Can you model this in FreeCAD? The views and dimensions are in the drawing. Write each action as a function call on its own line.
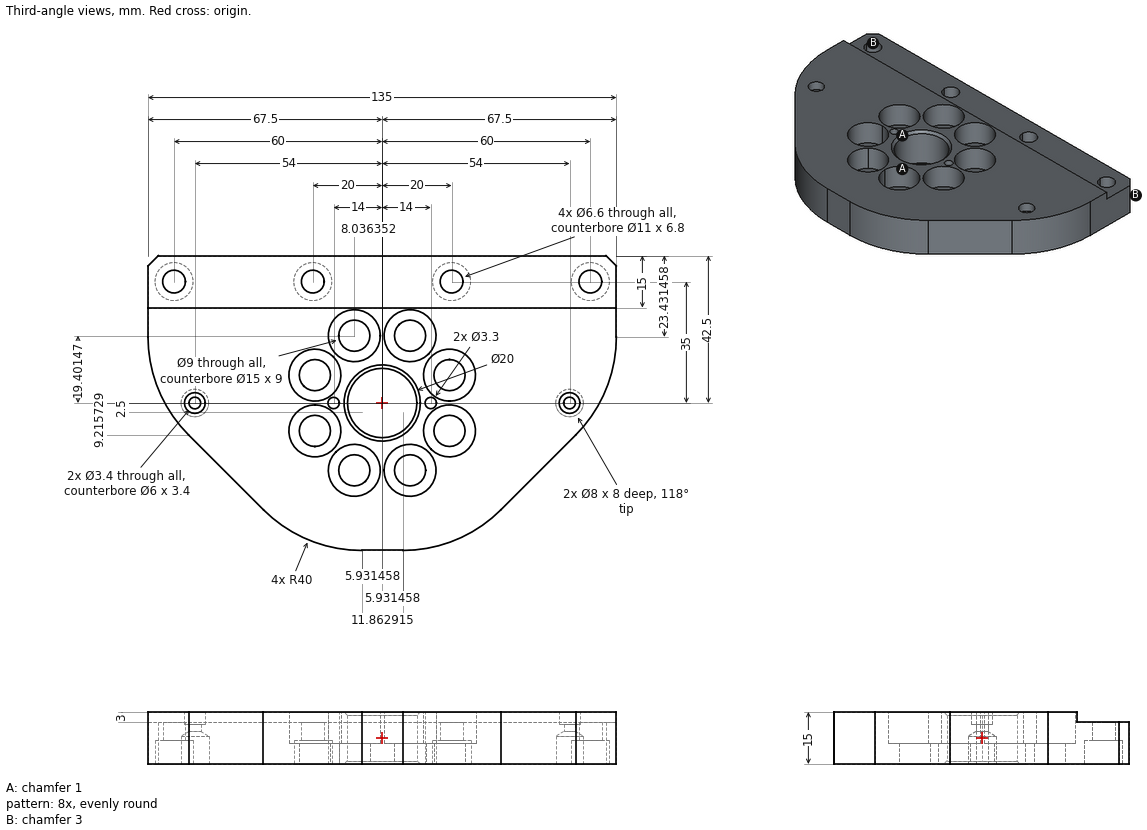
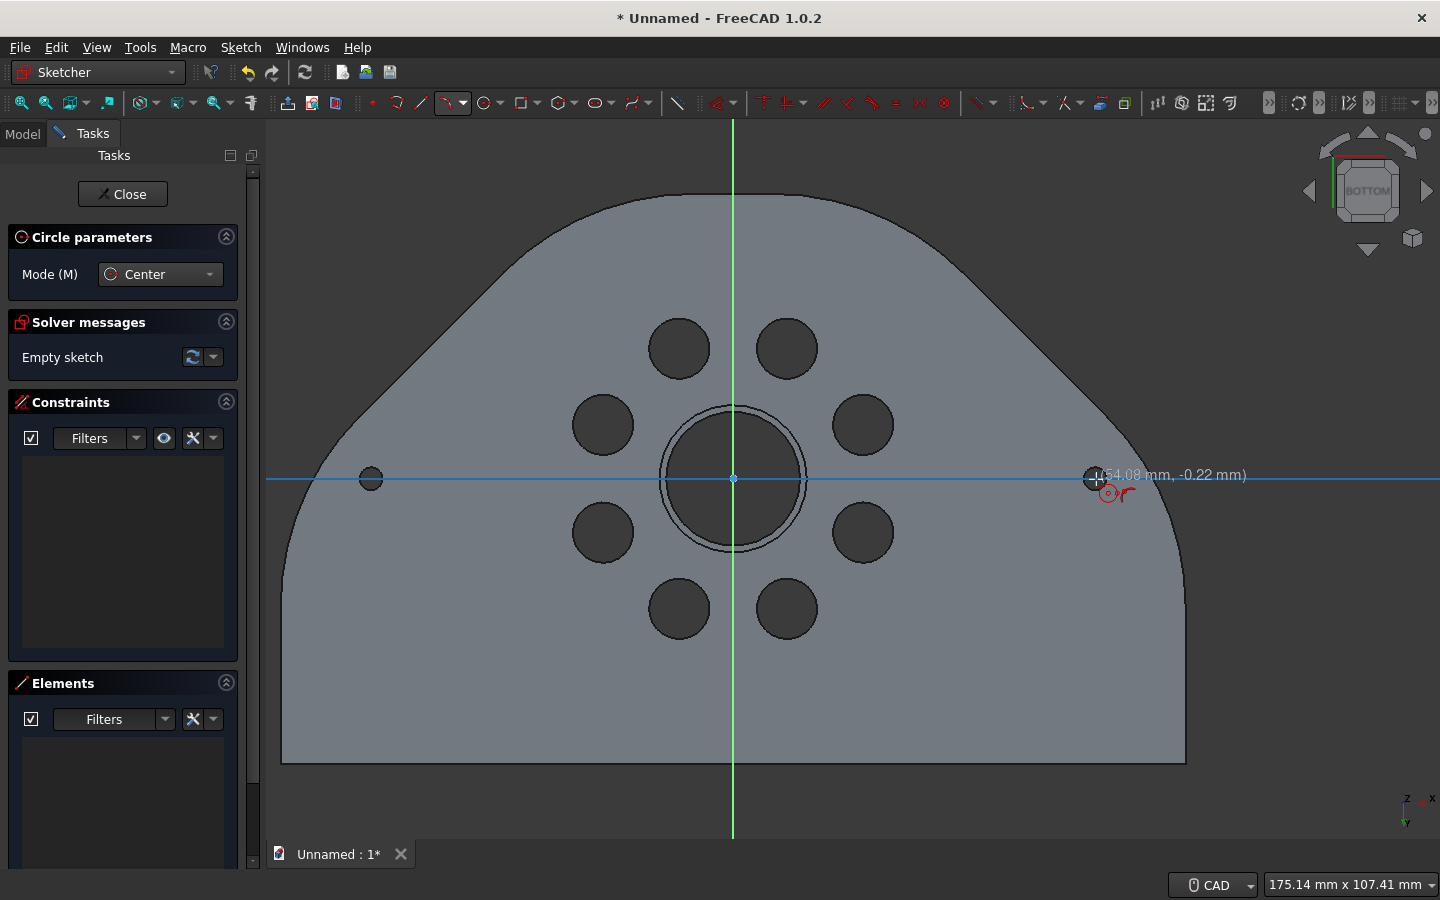
click(1095, 479)
move(1114, 460)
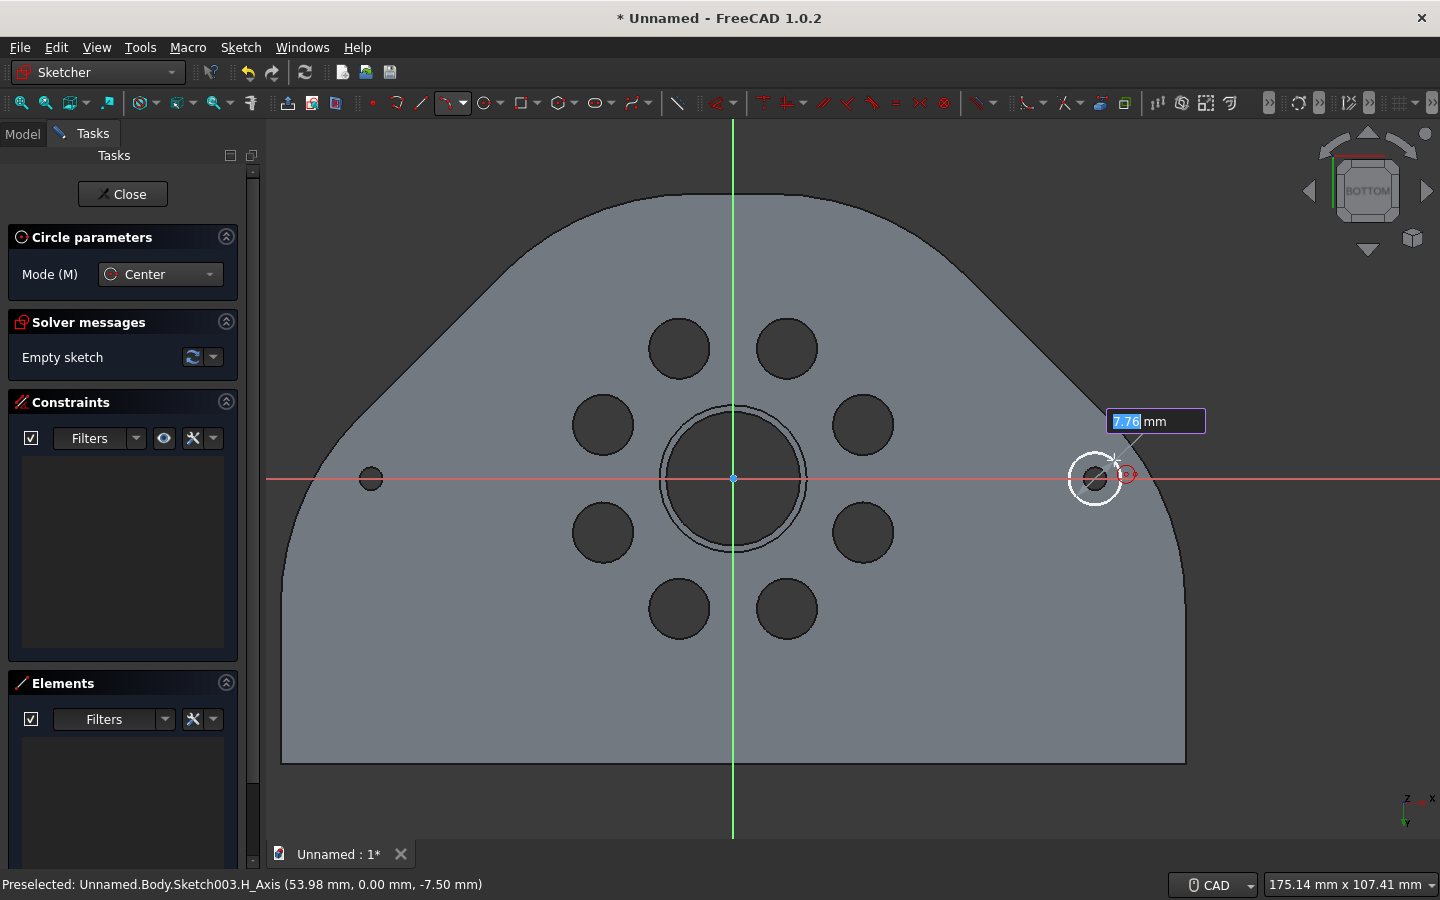
text(8)
key(Return)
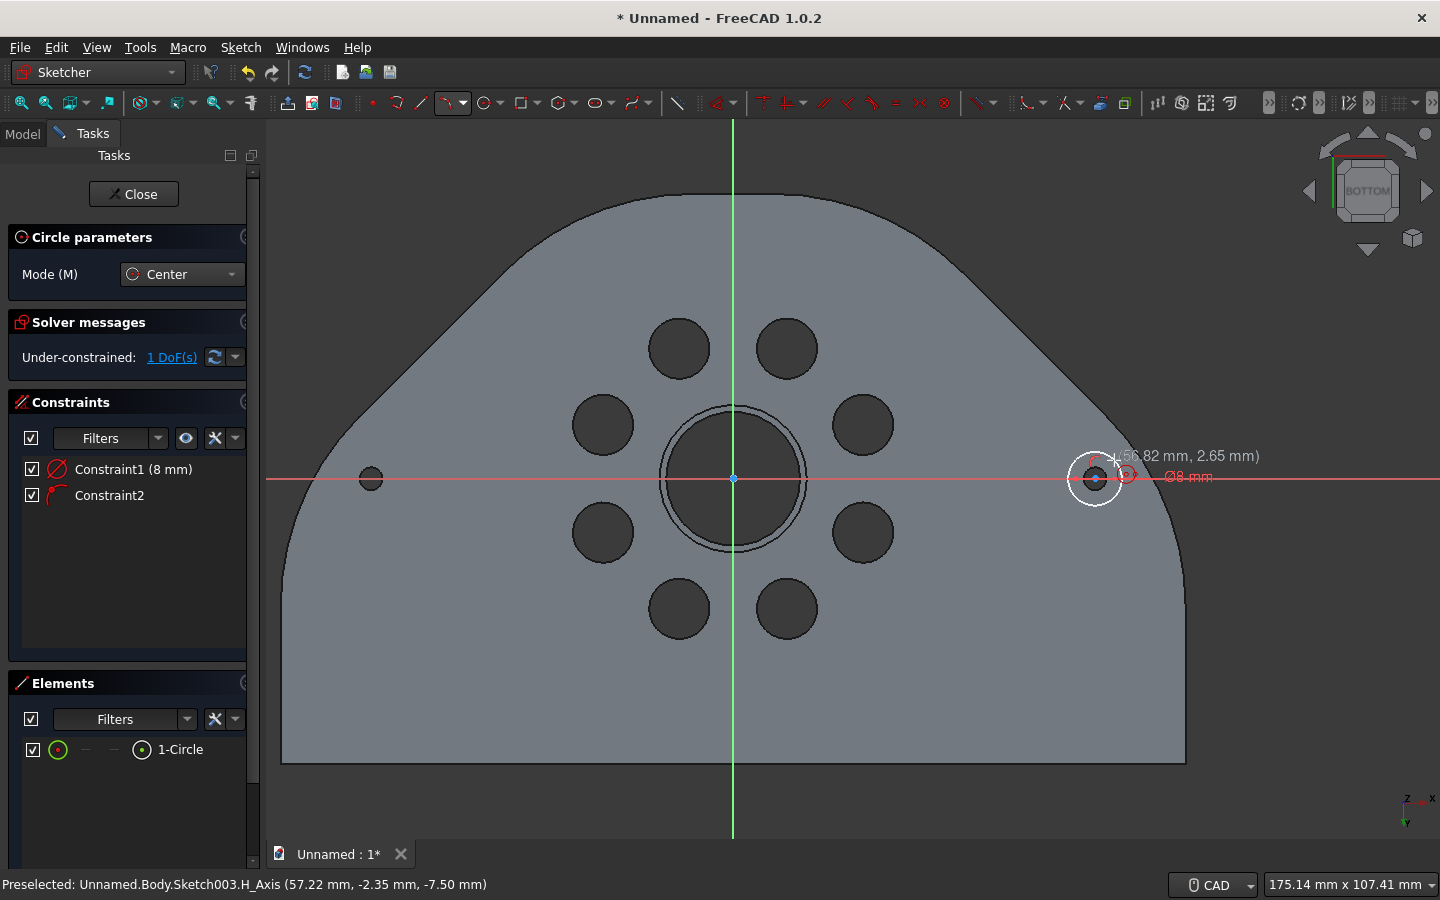
click(371, 479)
move(390, 460)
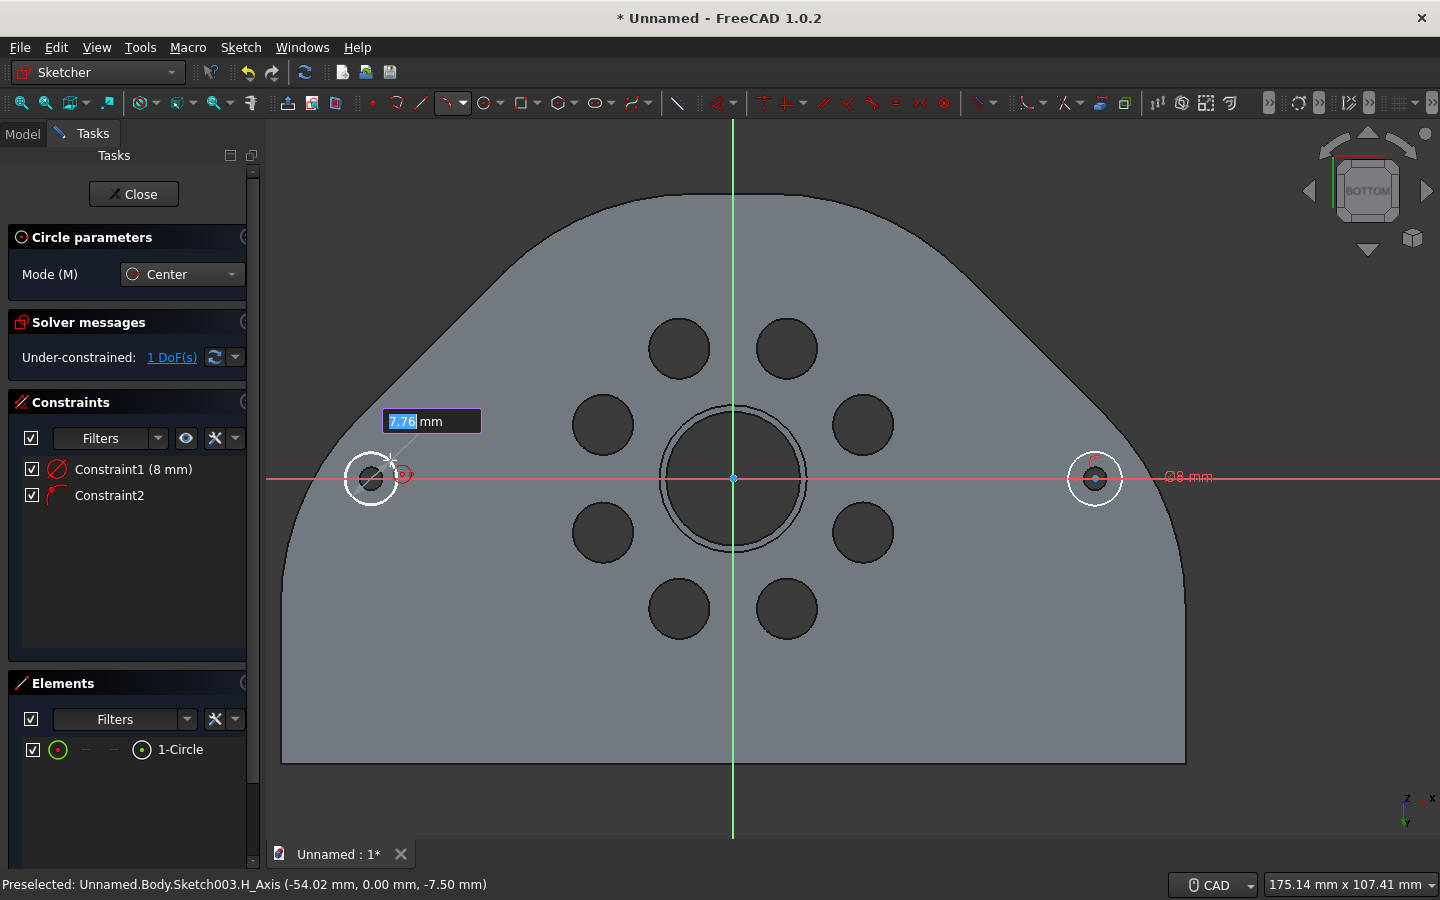
text(8)
key(Return)
key(Escape)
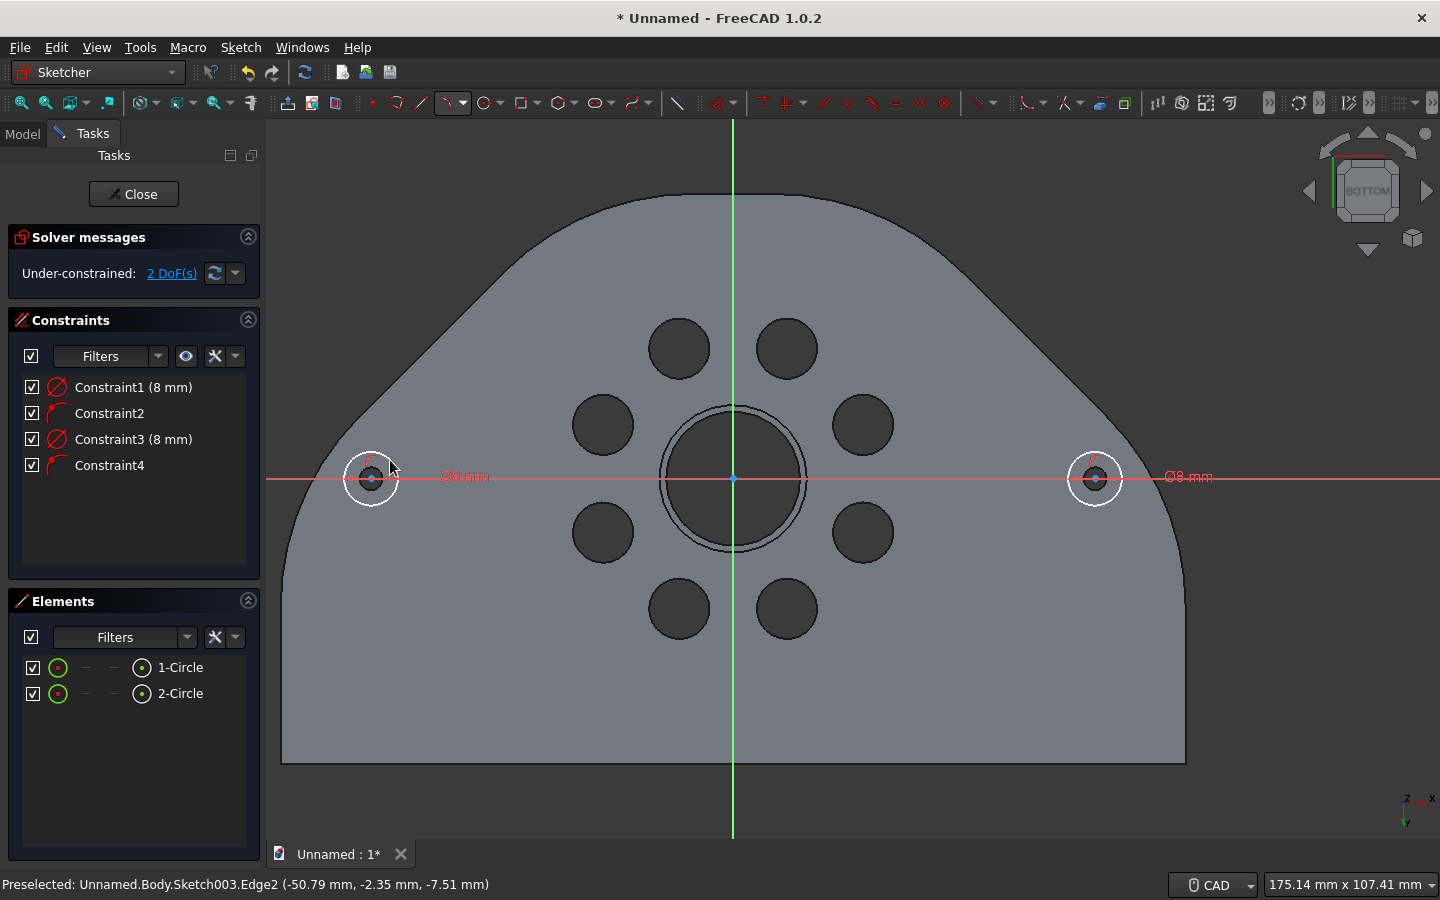
click(716, 104)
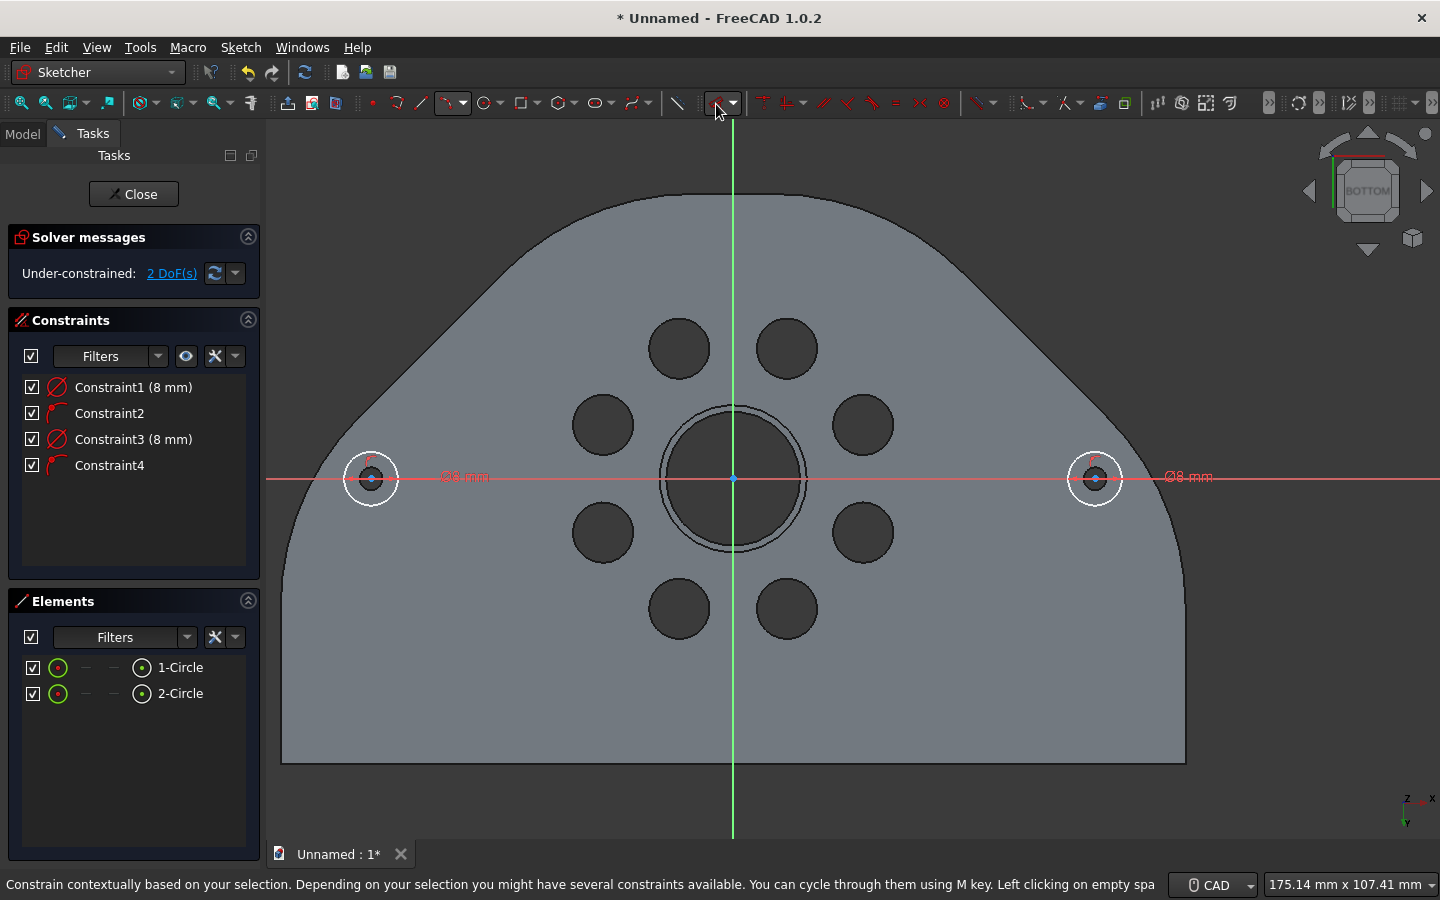
click(1095, 479)
click(914, 513)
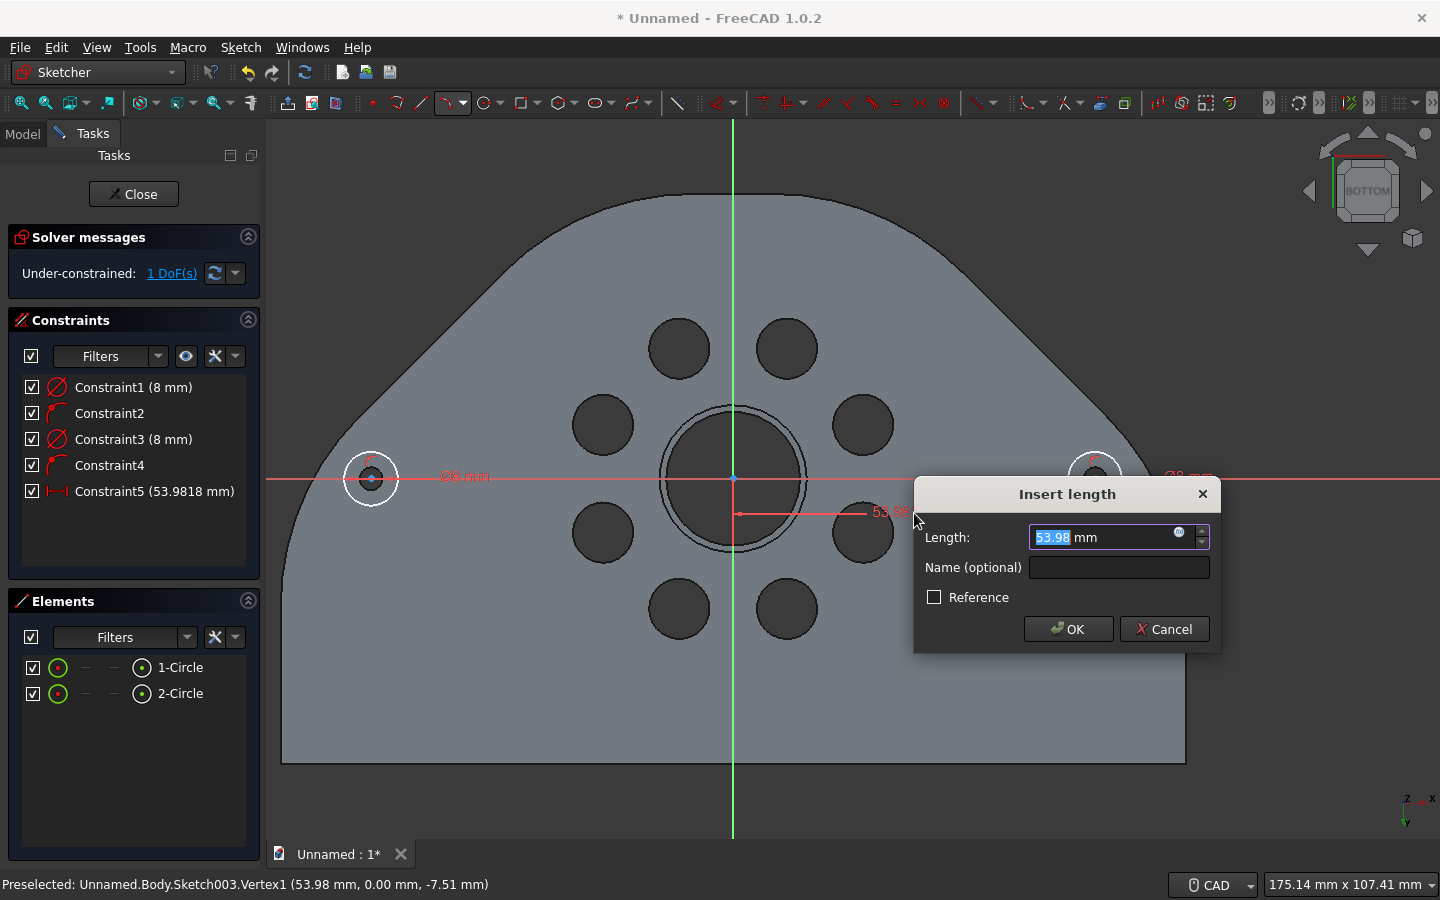
text(54)
key(Return)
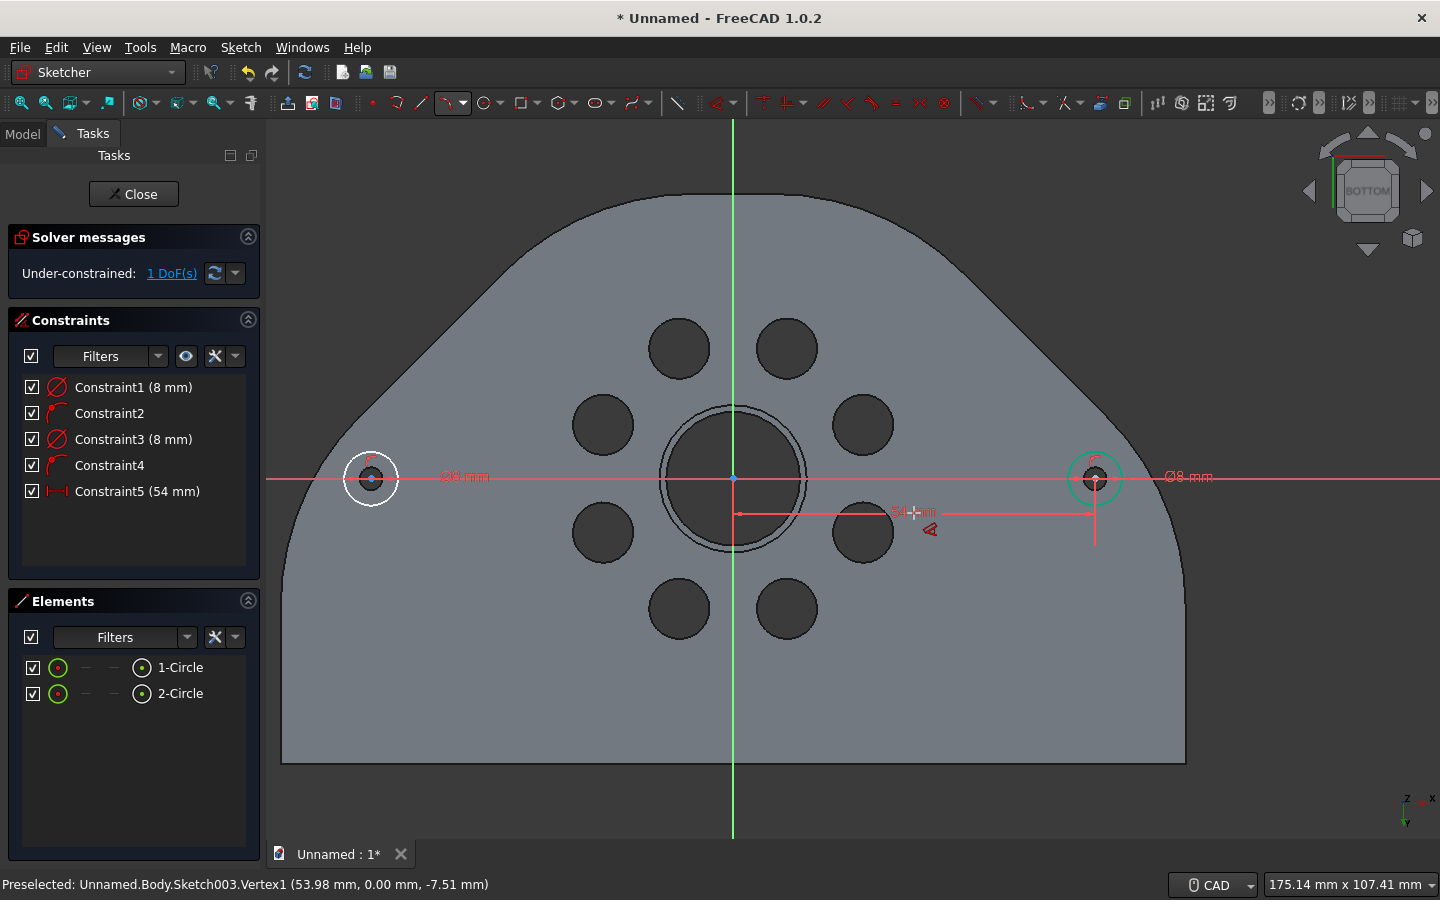
click(371, 479)
click(552, 513)